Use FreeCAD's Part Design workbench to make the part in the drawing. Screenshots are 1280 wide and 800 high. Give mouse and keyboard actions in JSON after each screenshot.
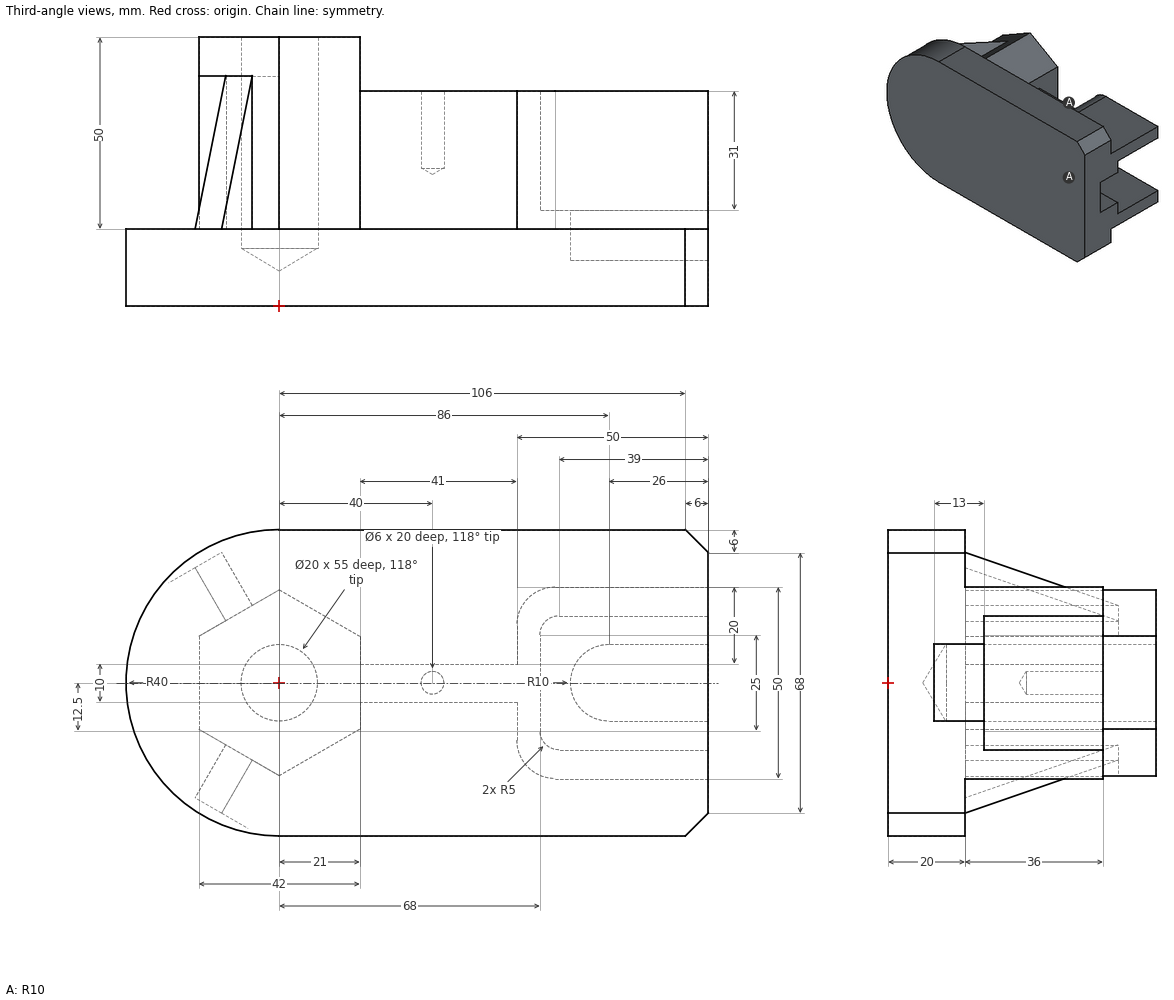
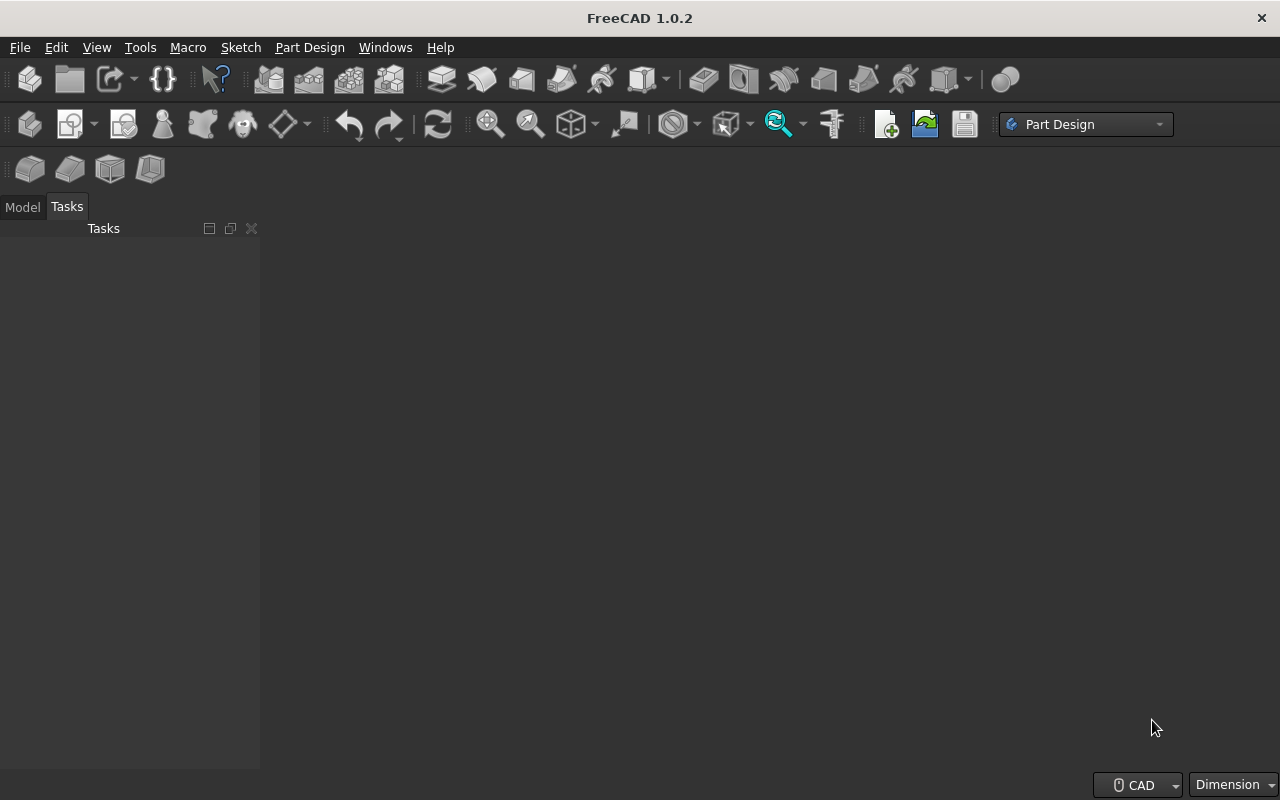
{"action": "left_click", "coordinate": [886, 124]}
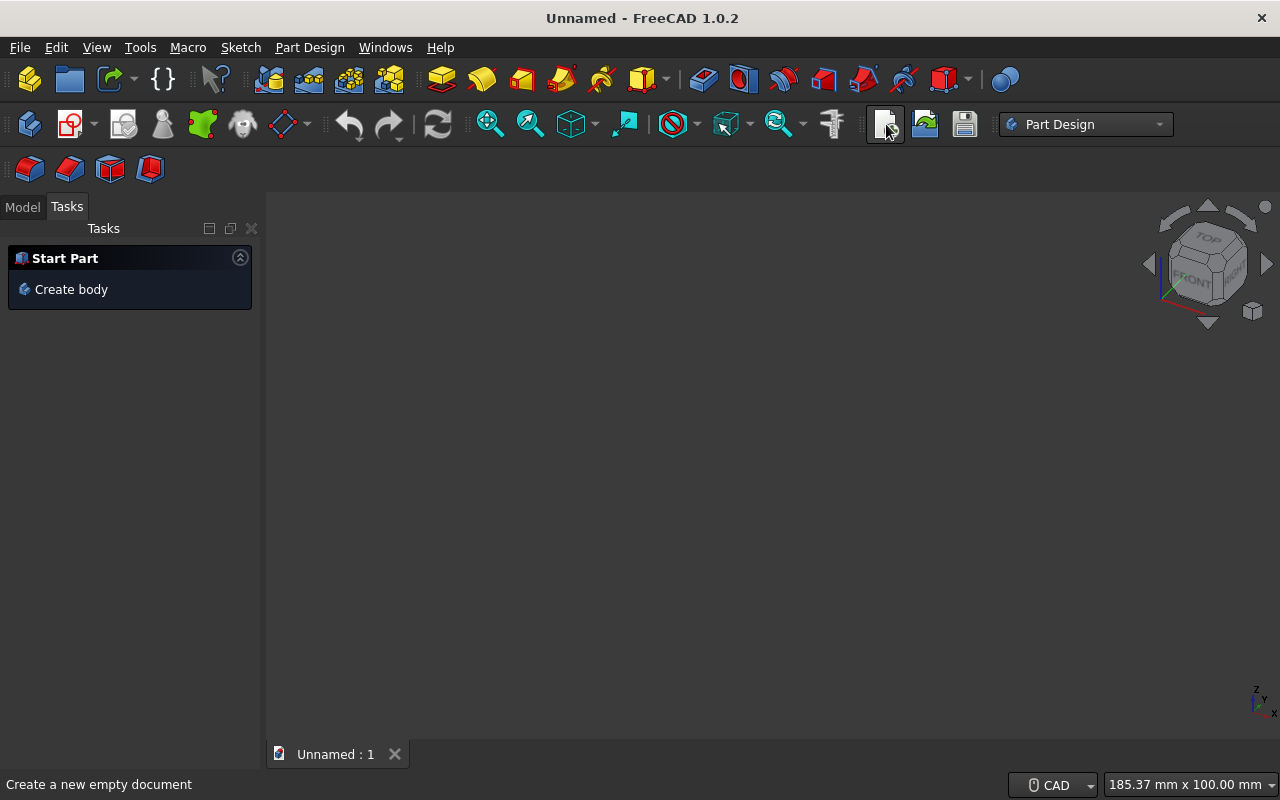
{"action": "left_click", "coordinate": [70, 124]}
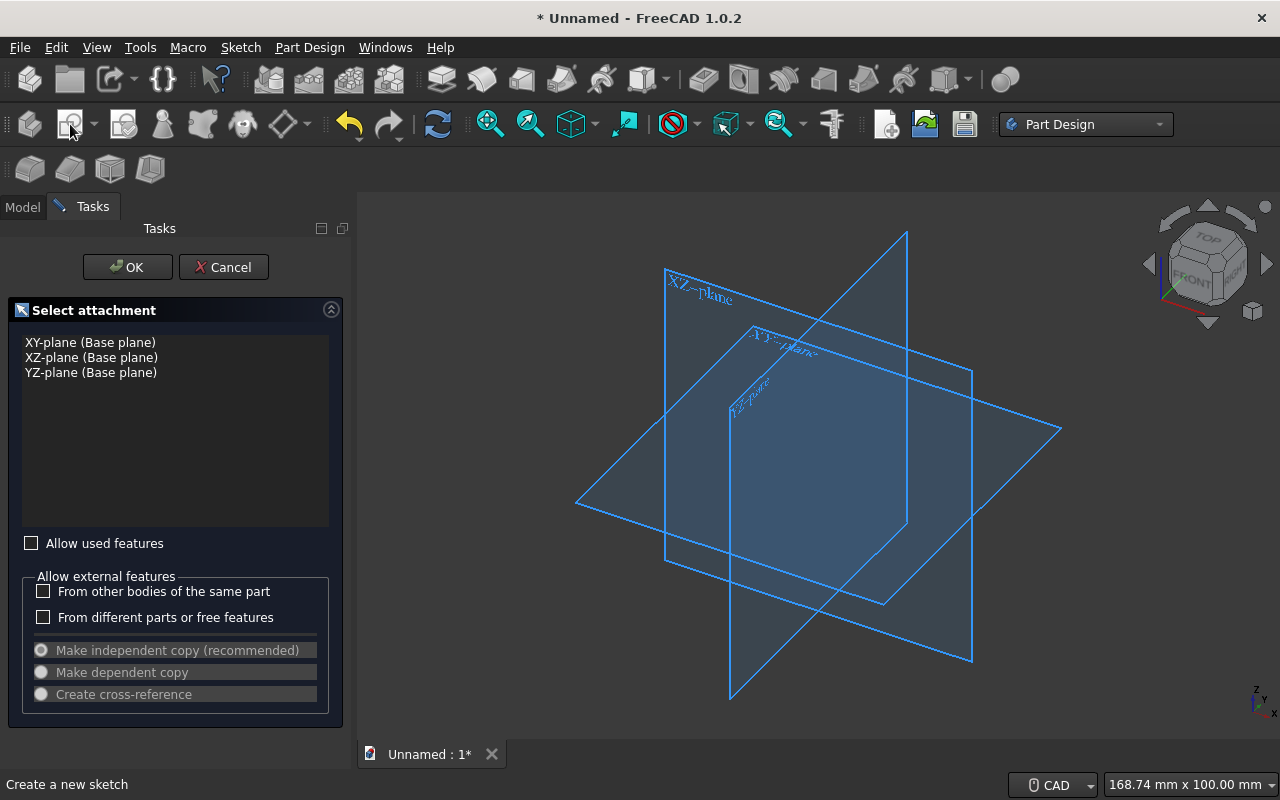
{"action": "left_click", "coordinate": [82, 358]}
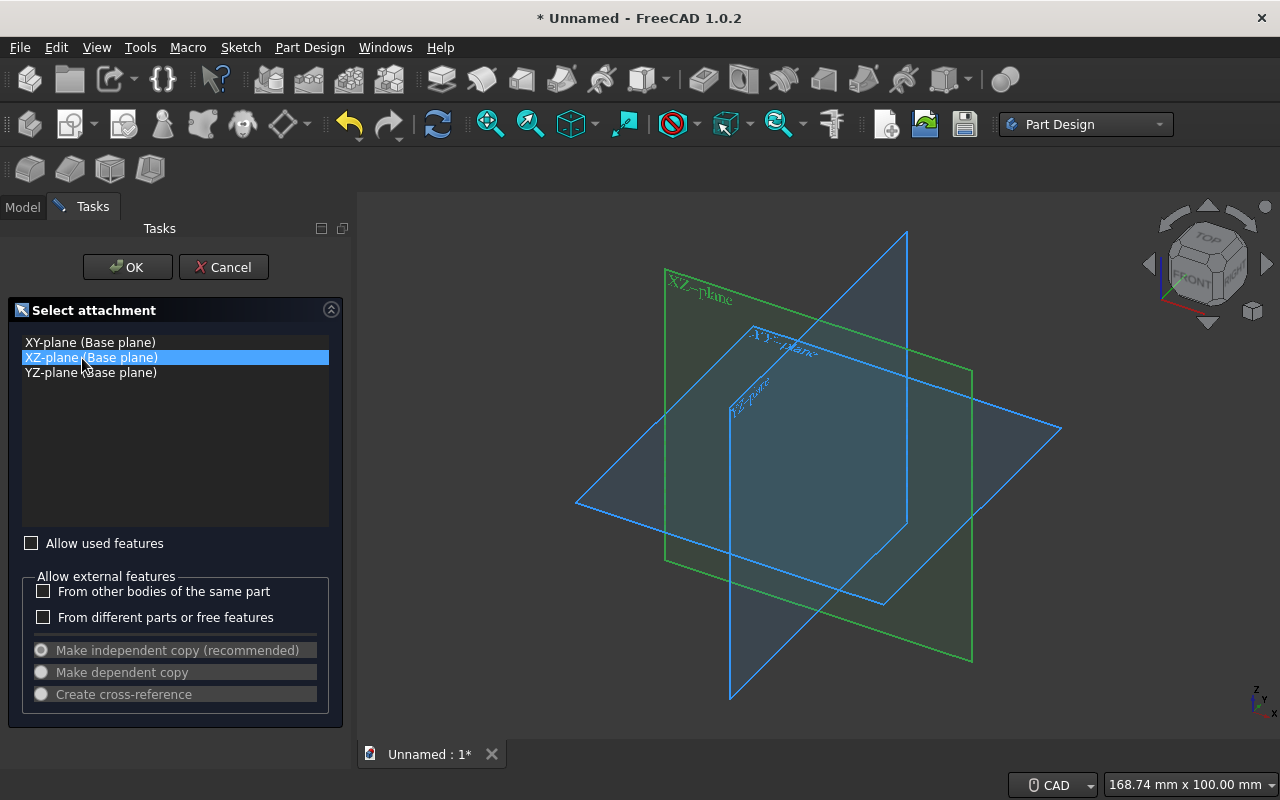
{"action": "left_click", "coordinate": [128, 267]}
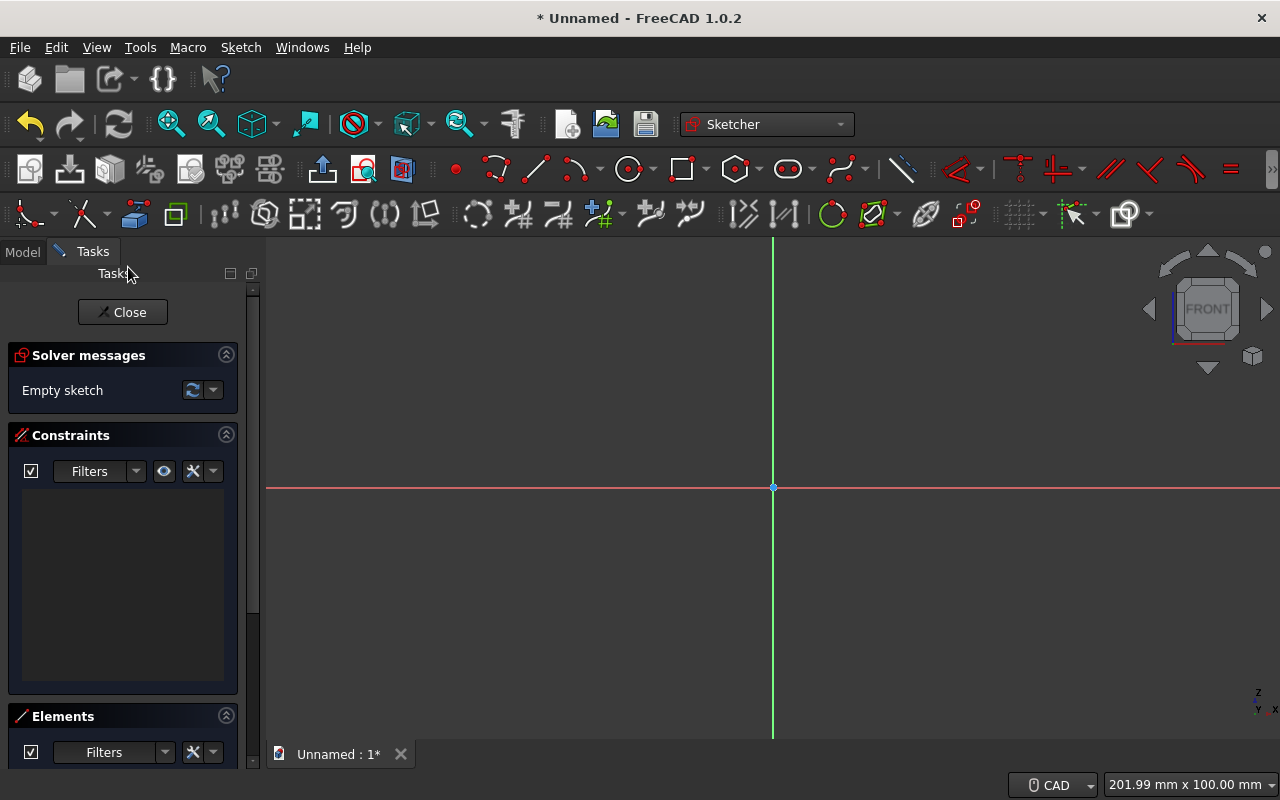
{"action": "scroll", "coordinate": [294, 488], "scroll_direction": "down", "scroll_amount": 2}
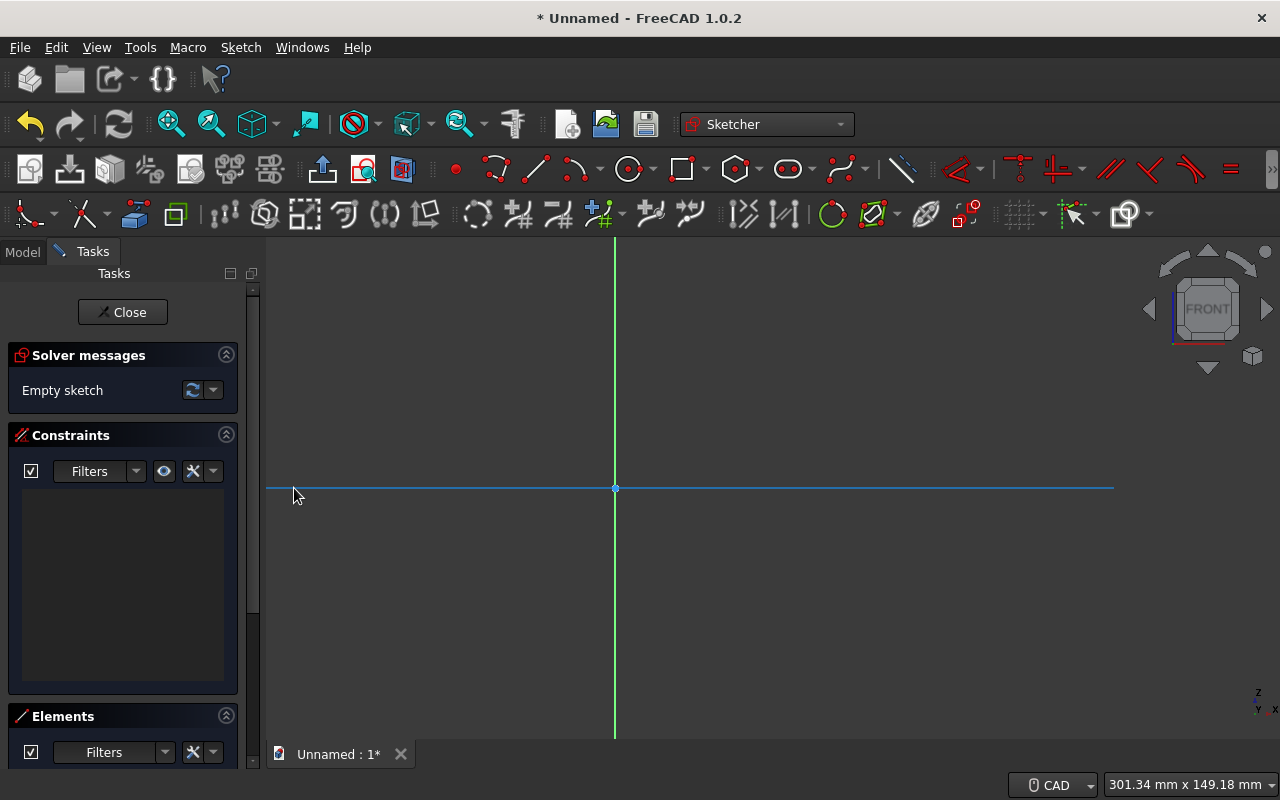
{"action": "left_click", "coordinate": [496, 170]}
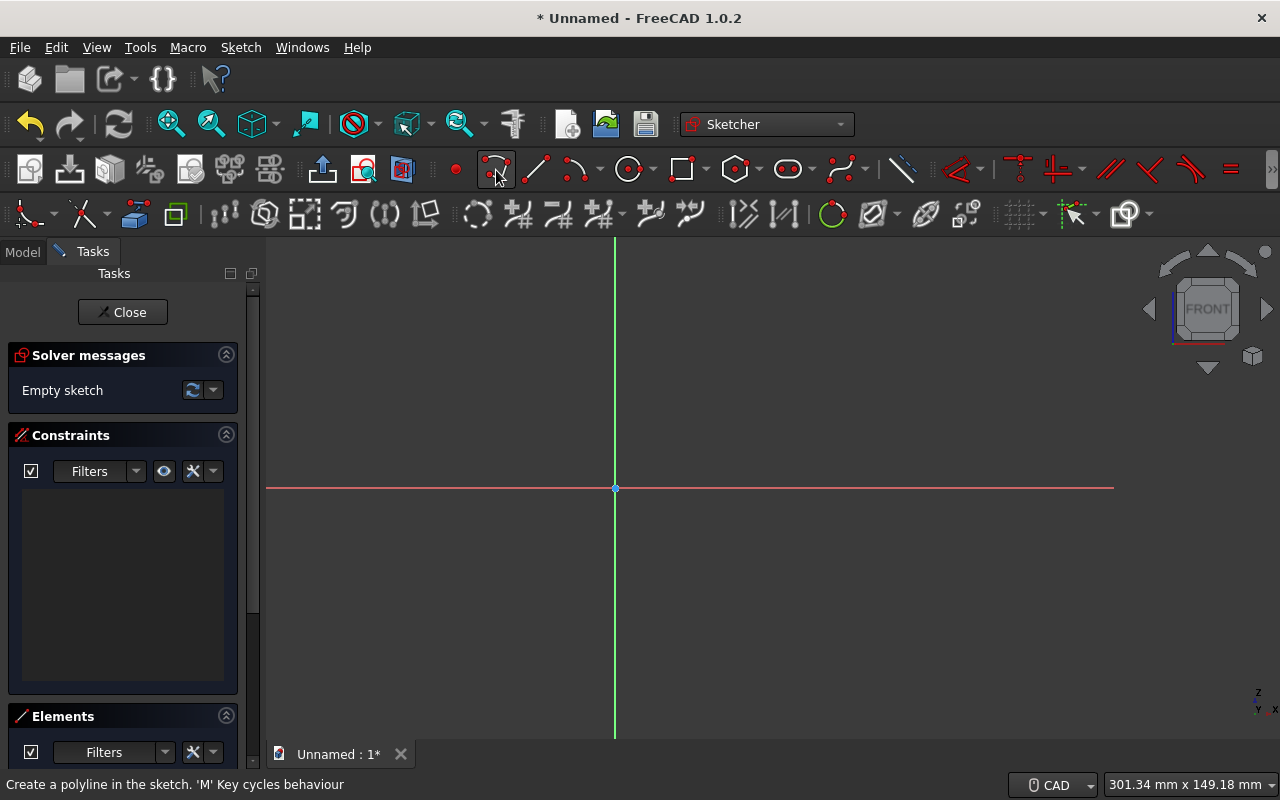
{"action": "left_click", "coordinate": [615, 354]}
{"action": "left_click", "coordinate": [972, 354]}
{"action": "left_click", "coordinate": [992, 374]}
{"action": "left_click", "coordinate": [992, 603]}
{"action": "left_click", "coordinate": [972, 623]}
{"action": "left_click", "coordinate": [615, 623]}
{"action": "right_click", "coordinate": [615, 623]}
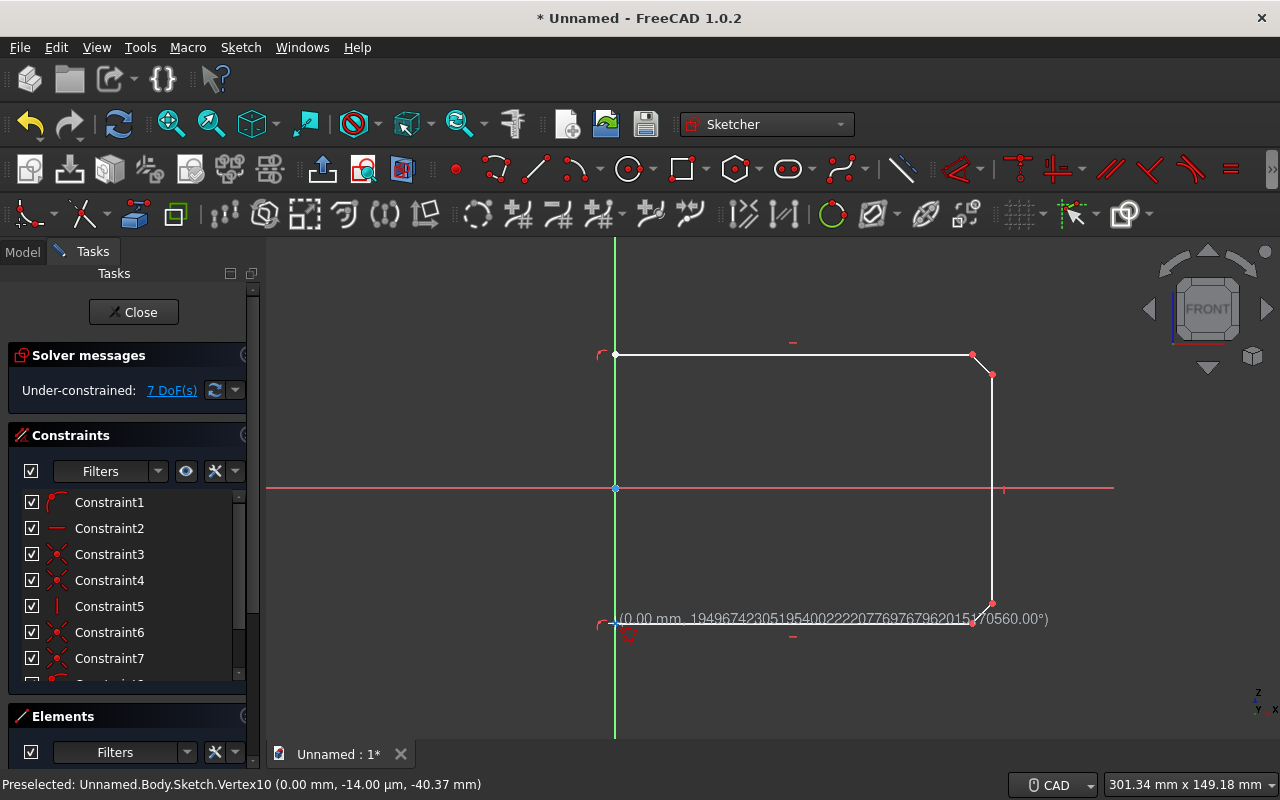
{"action": "left_click", "coordinate": [602, 170]}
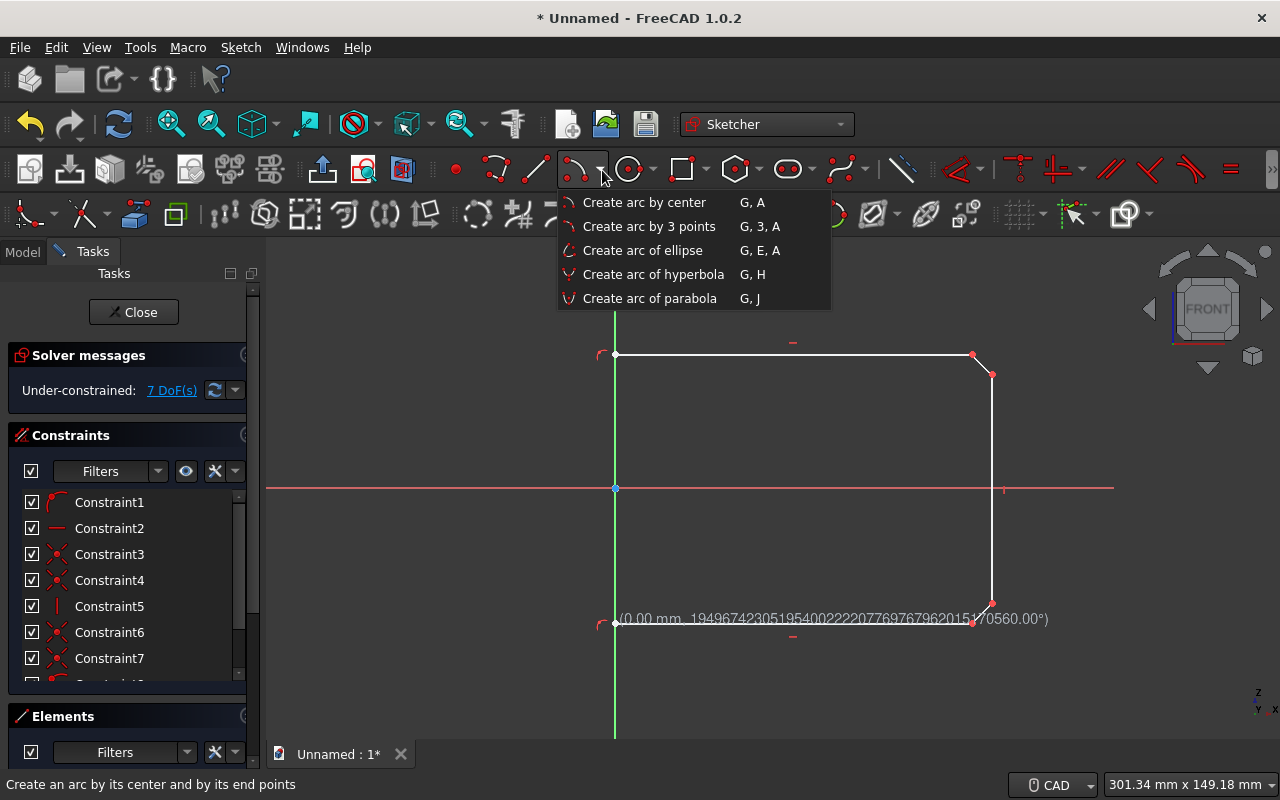
{"action": "left_click", "coordinate": [694, 226]}